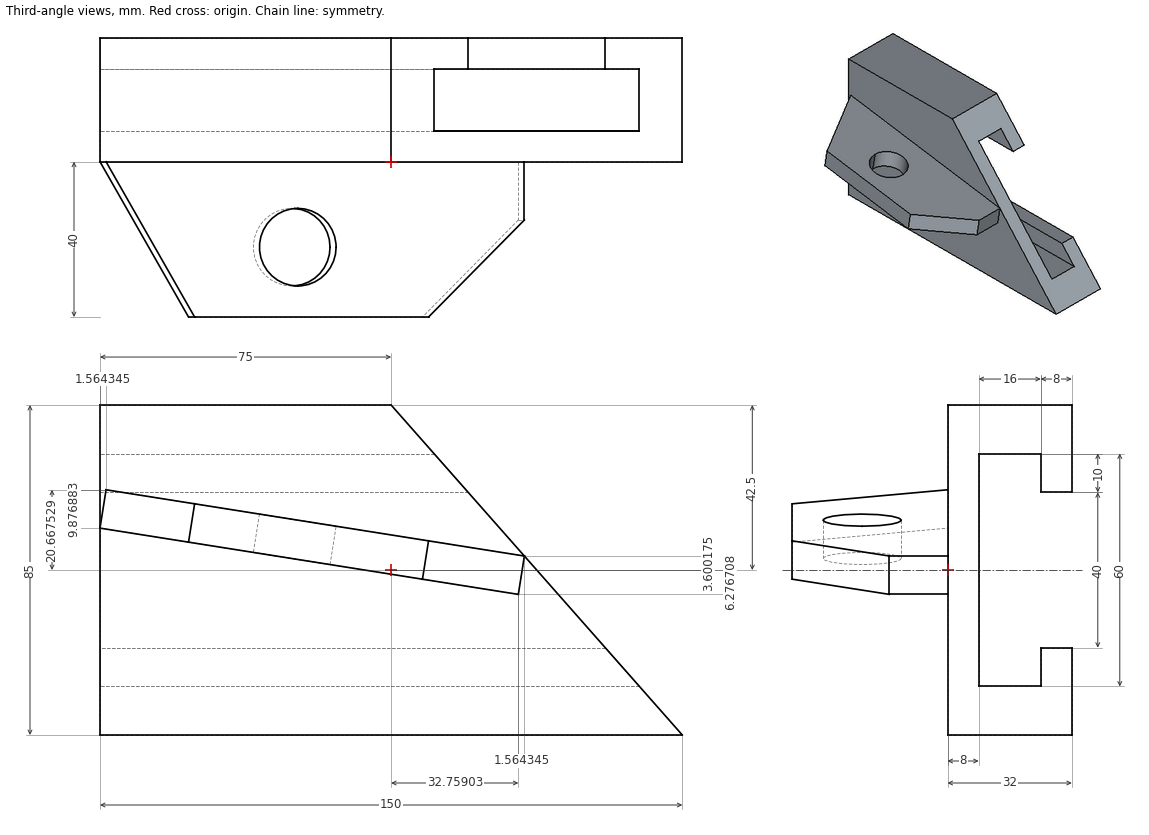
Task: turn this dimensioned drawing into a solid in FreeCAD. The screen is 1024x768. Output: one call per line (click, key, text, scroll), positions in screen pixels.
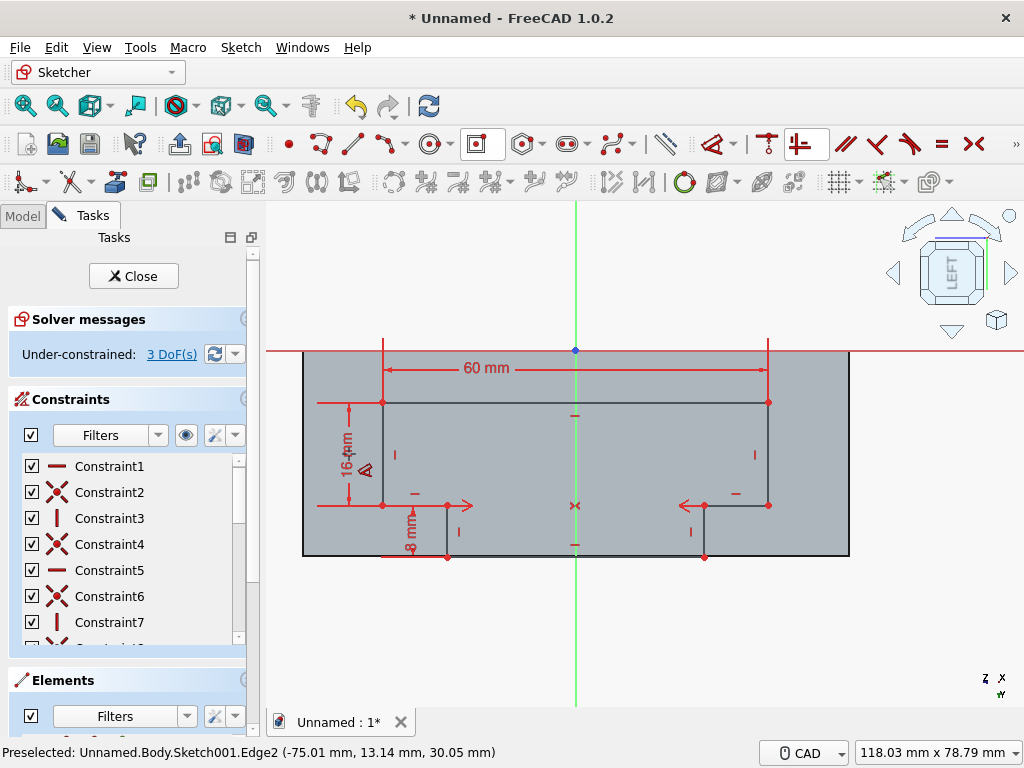
click(402, 506)
click(430, 472)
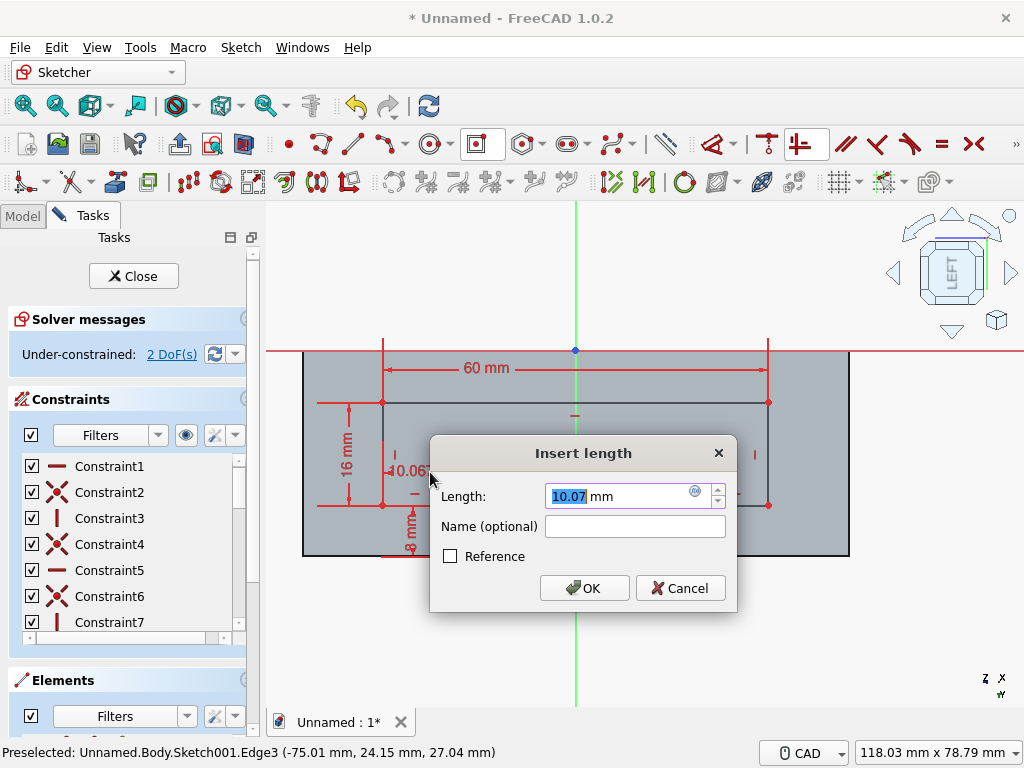
text(10)
key(Return)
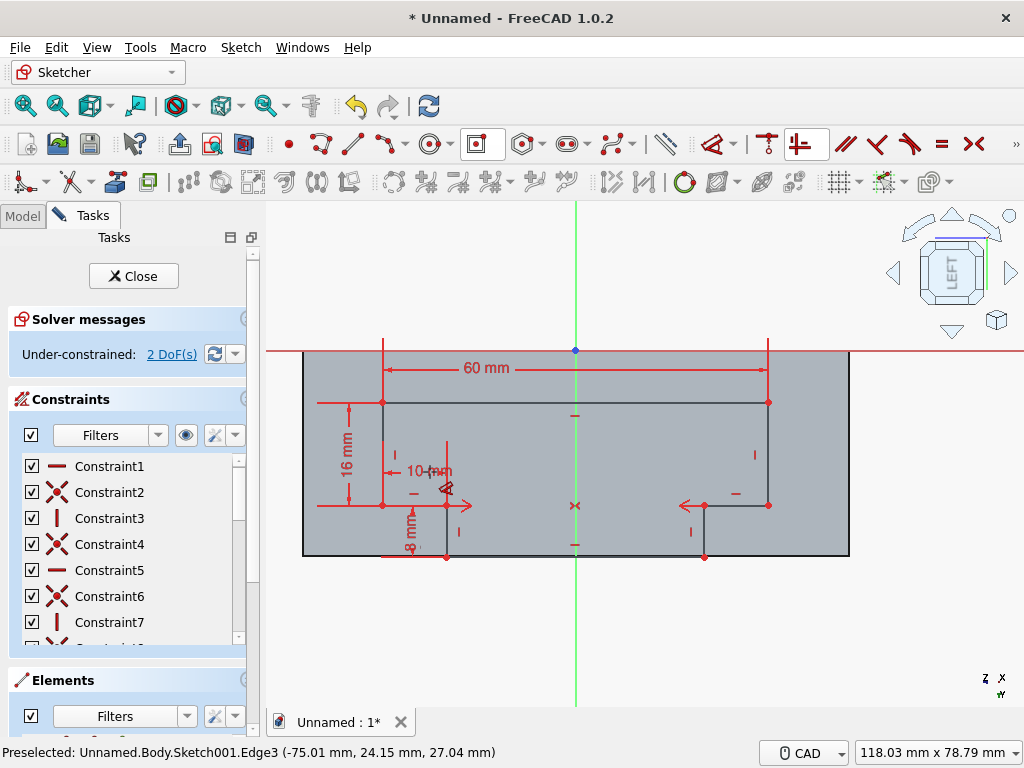
click(524, 557)
click(516, 591)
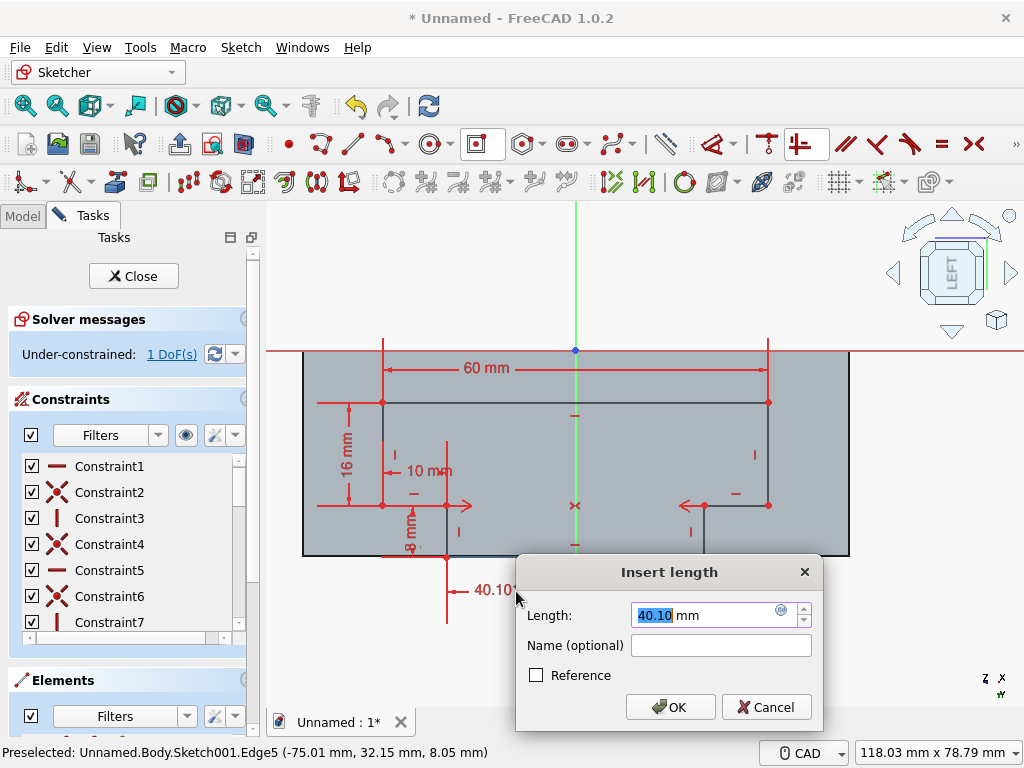
text(40)
key(Return)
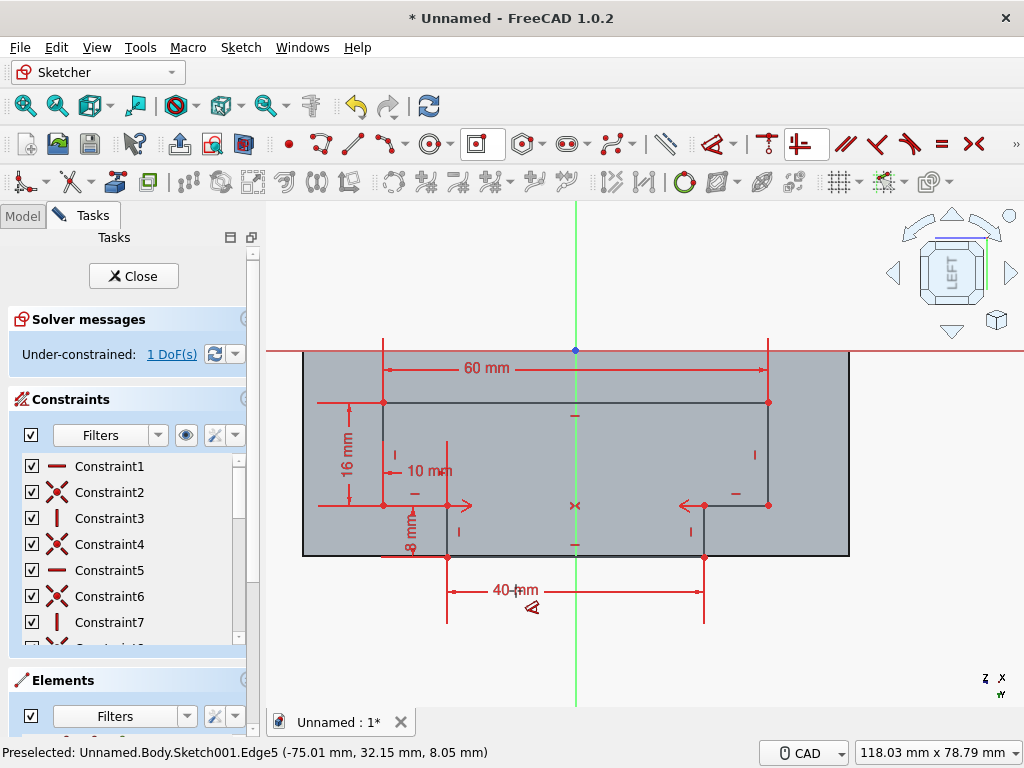
click(768, 403)
click(802, 377)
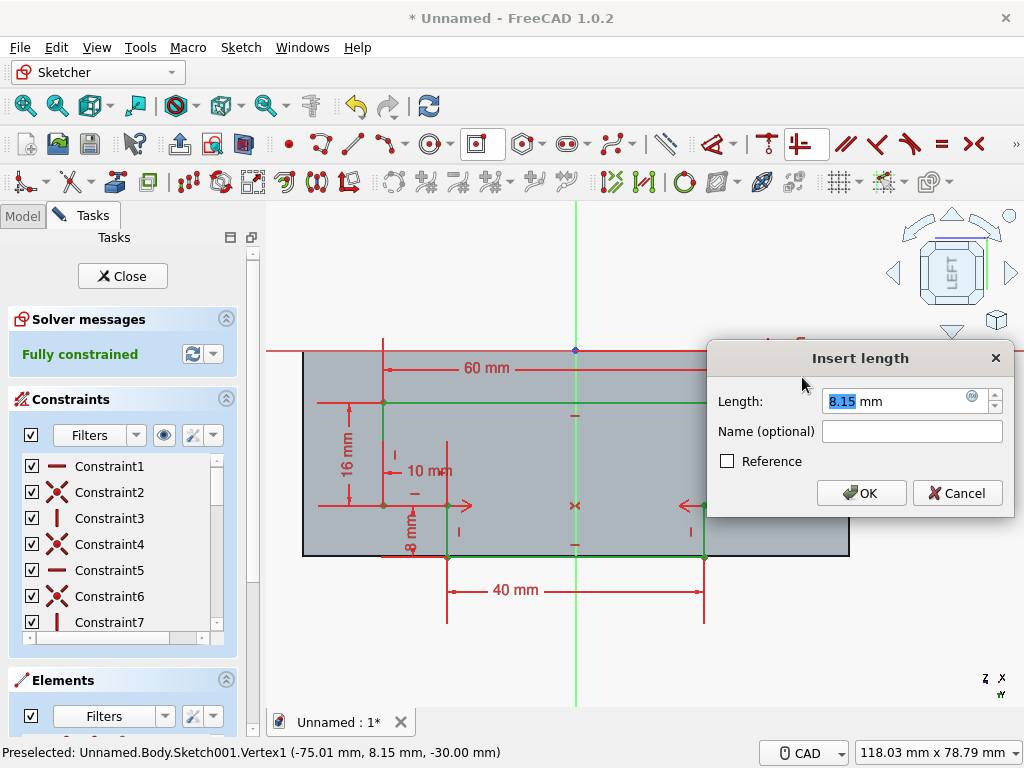
text(8)
key(Return)
key(Escape)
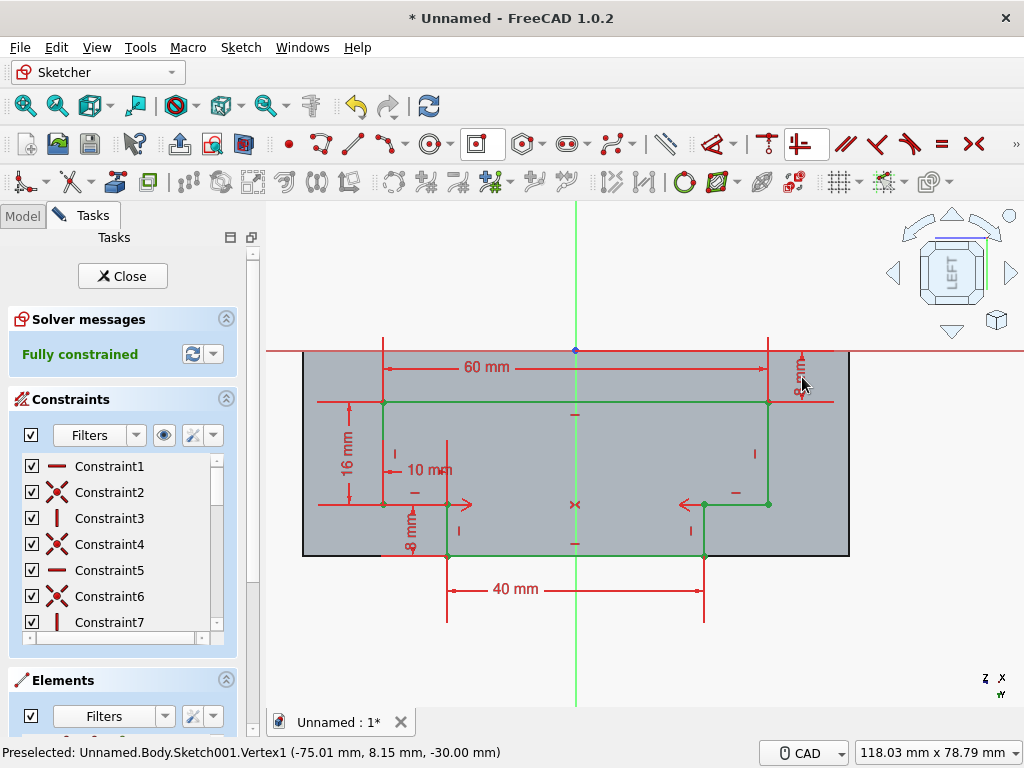
click(123, 276)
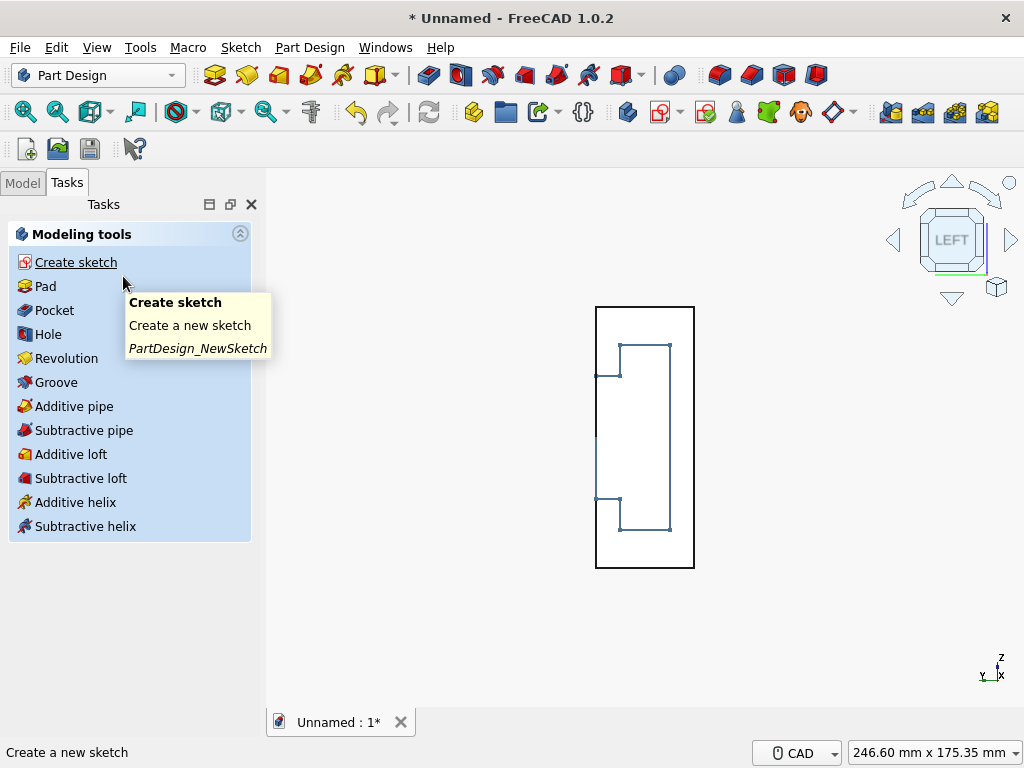
click(430, 76)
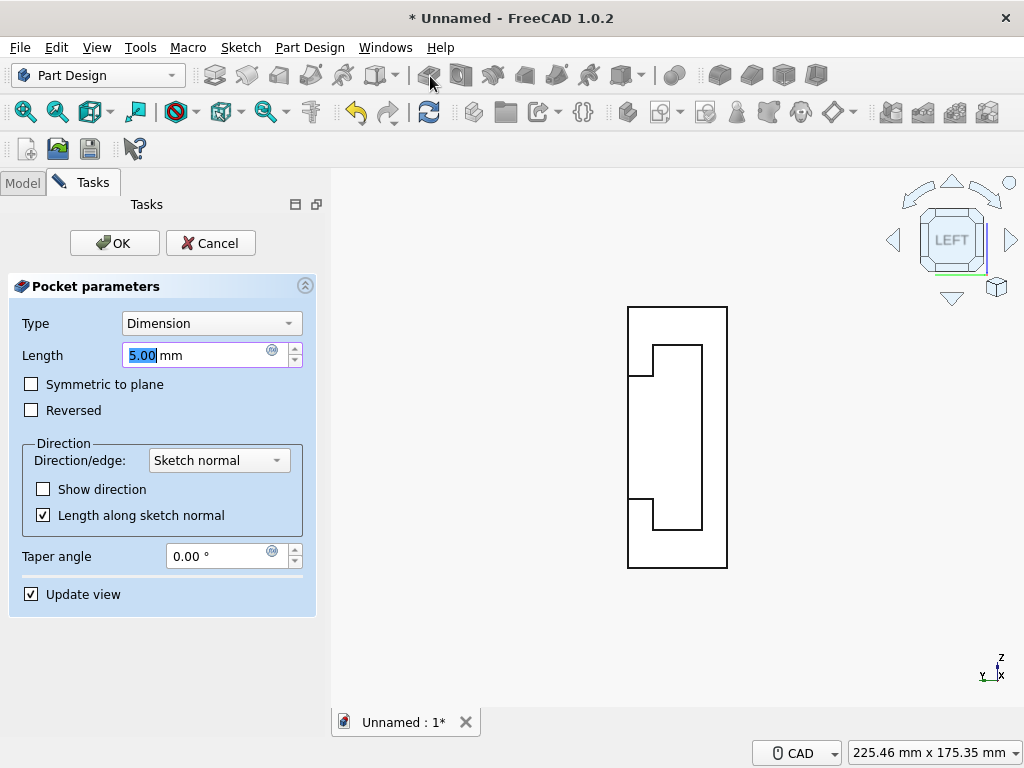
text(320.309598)
key(Tab)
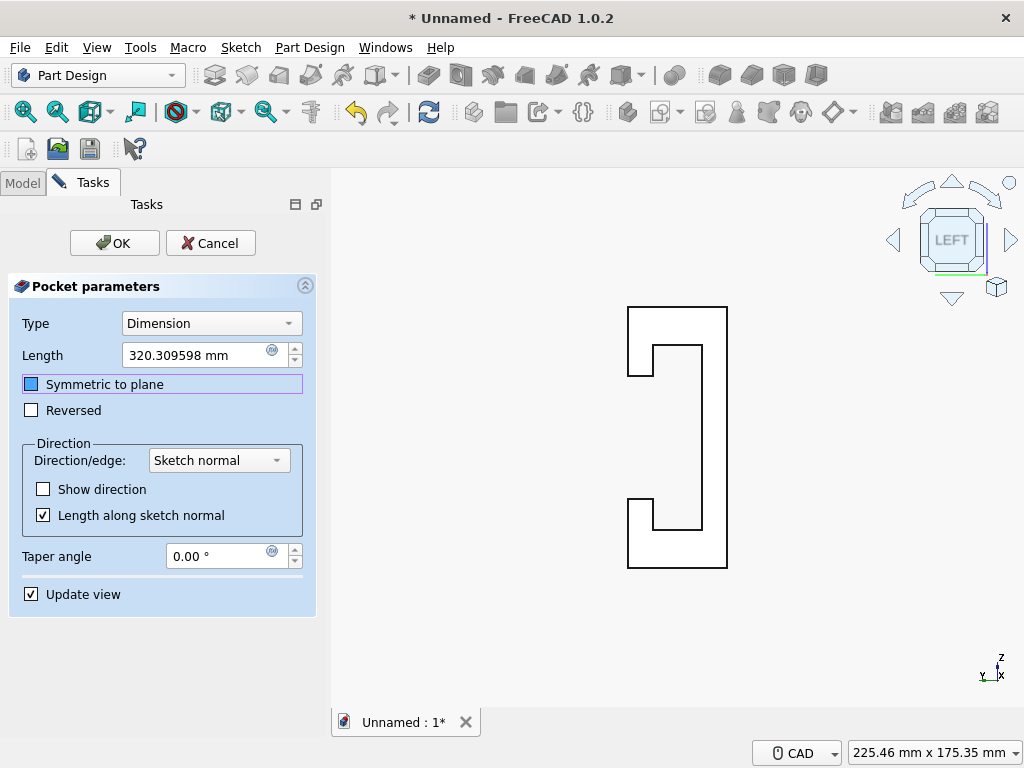
click(30, 384)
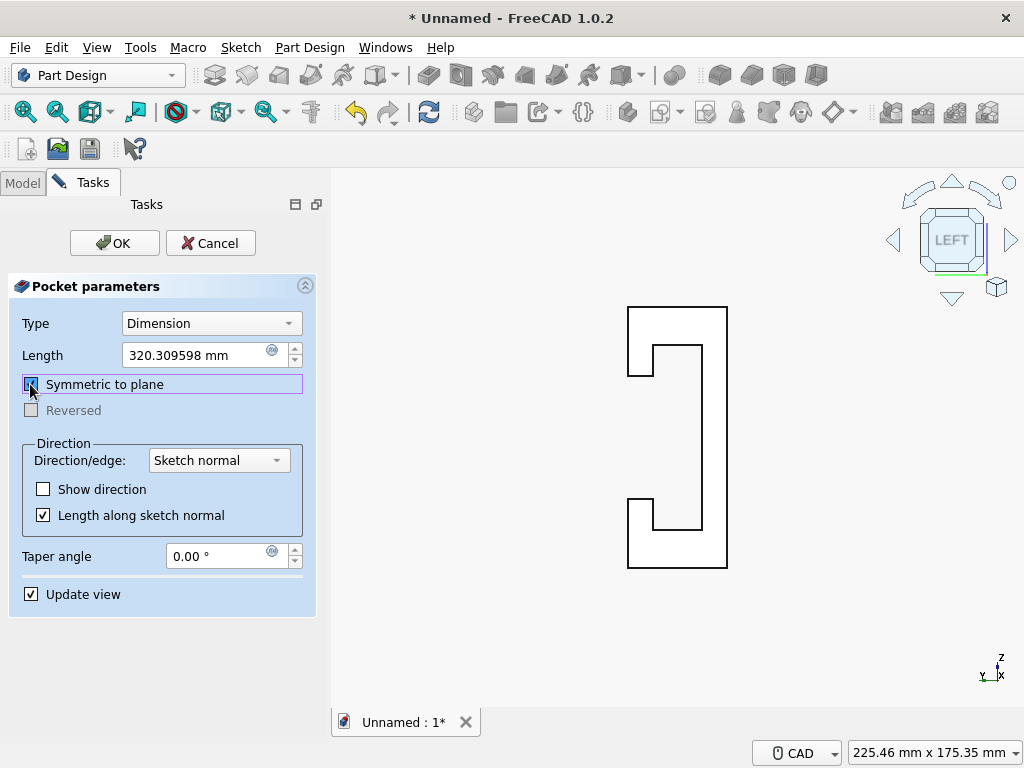
click(115, 243)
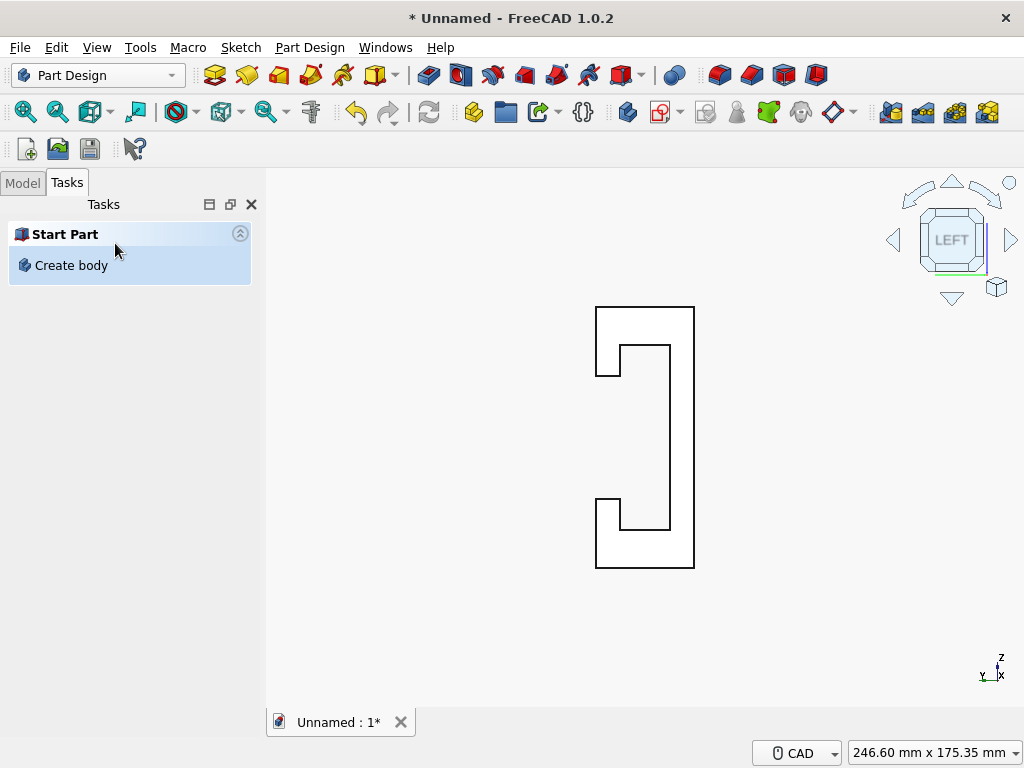
click(660, 112)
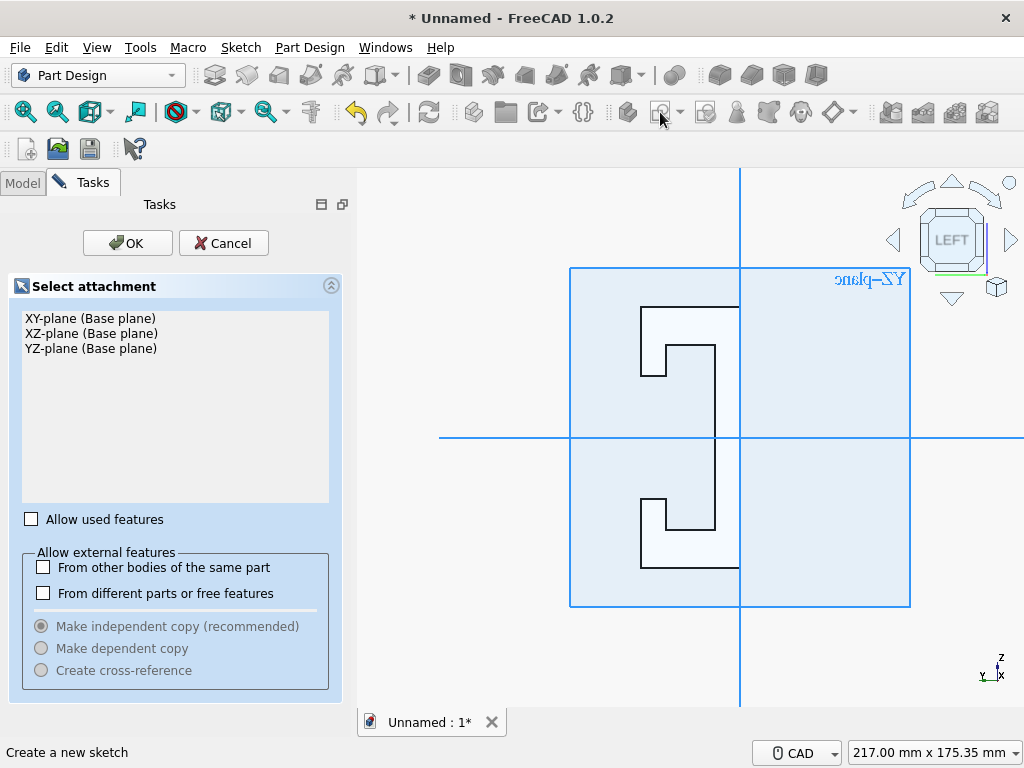
click(82, 334)